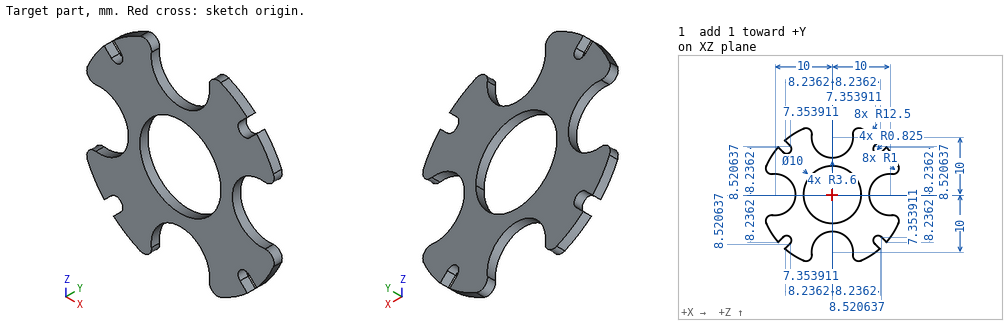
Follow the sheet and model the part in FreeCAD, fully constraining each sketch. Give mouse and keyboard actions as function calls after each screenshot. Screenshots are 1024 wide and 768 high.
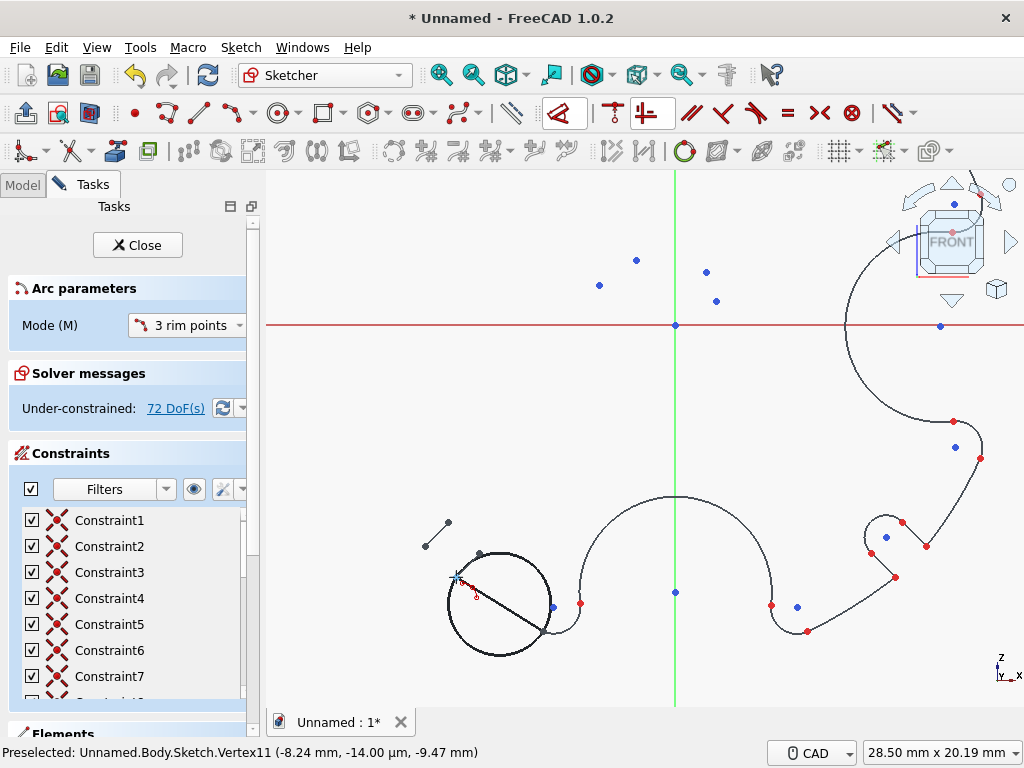
scroll(498, 606, up, 7)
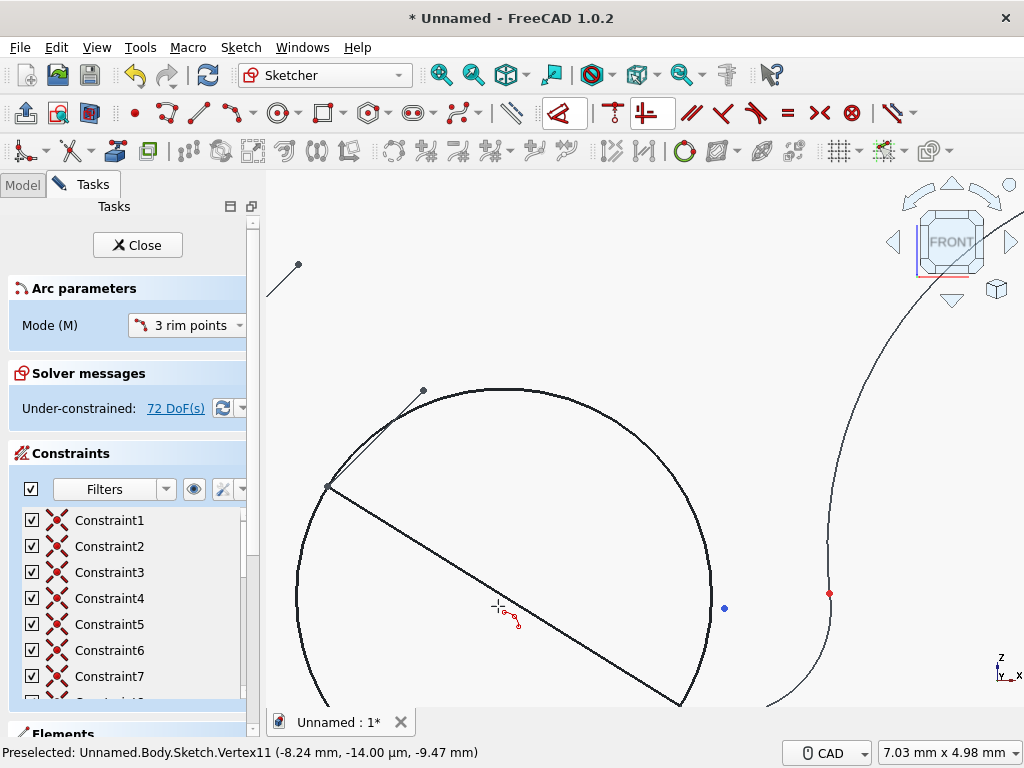
click(496, 605)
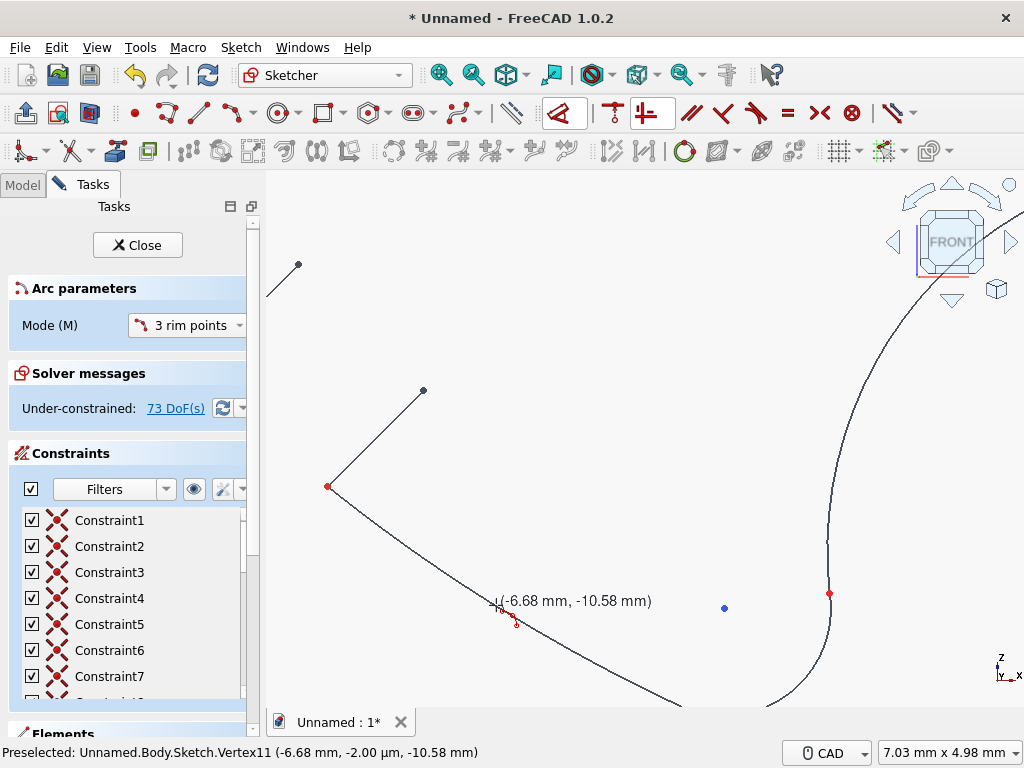
scroll(476, 591, down, 10)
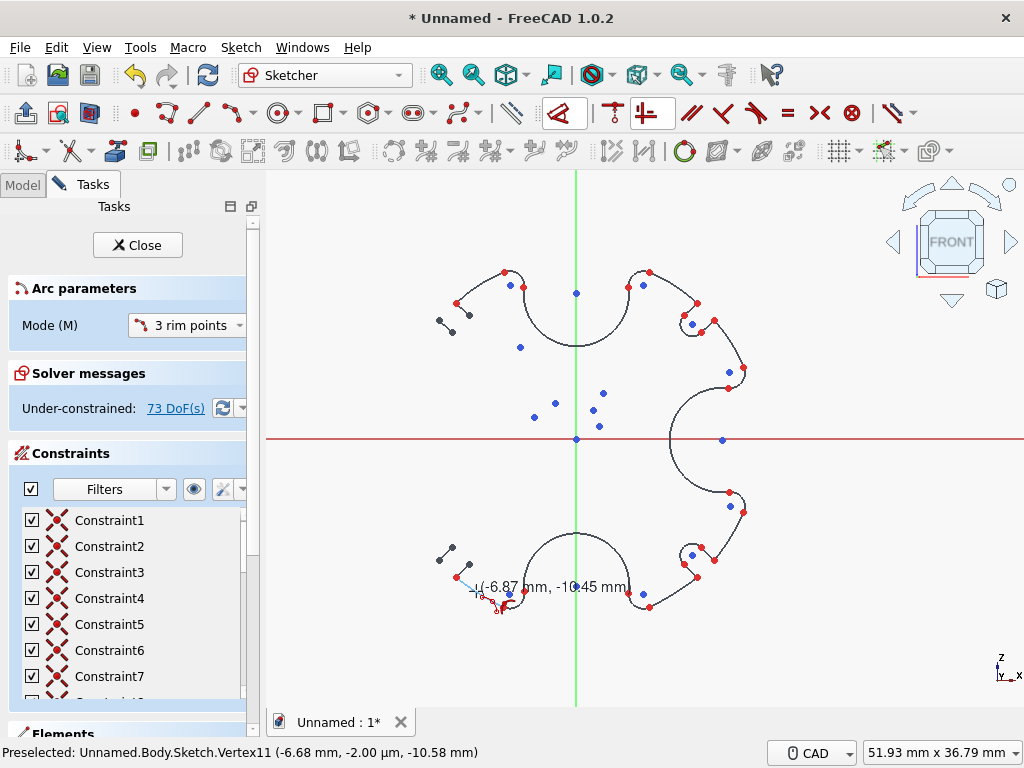
scroll(469, 564, up, 3)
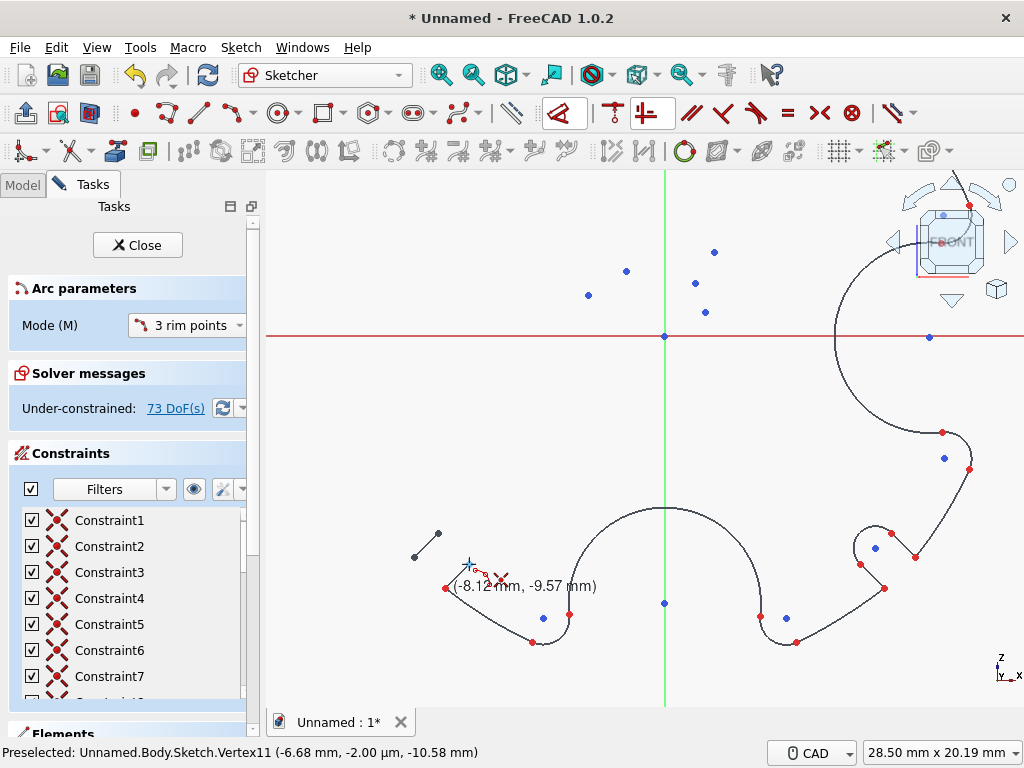
click(469, 564)
click(438, 533)
click(469, 532)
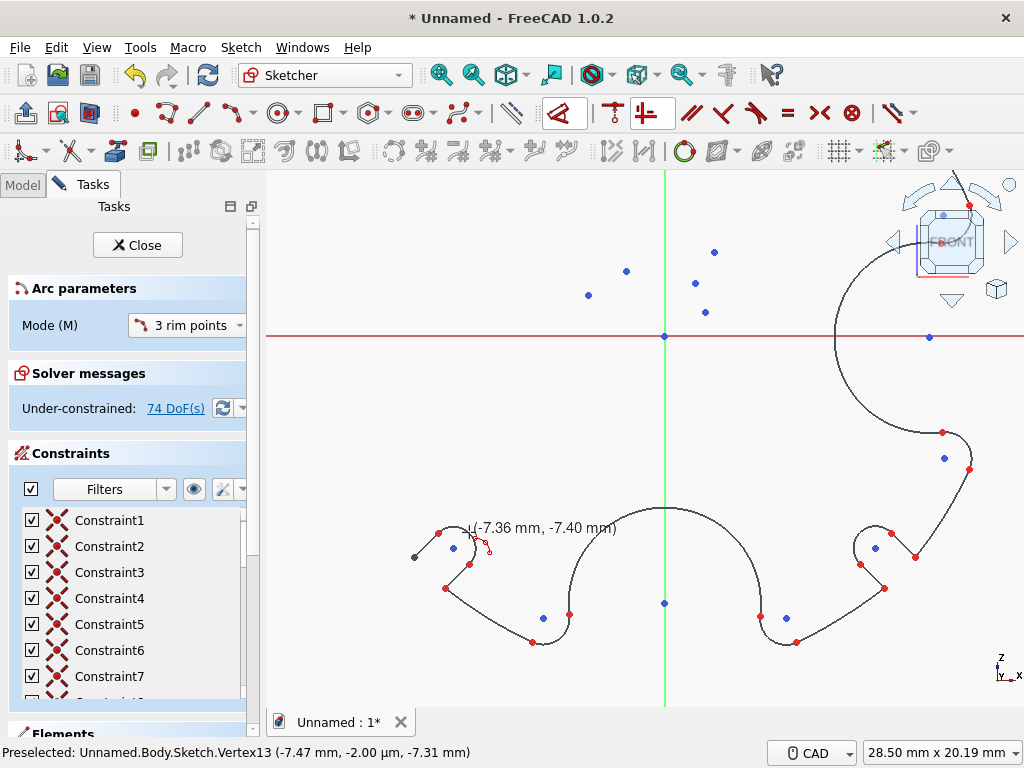
click(414, 557)
click(360, 468)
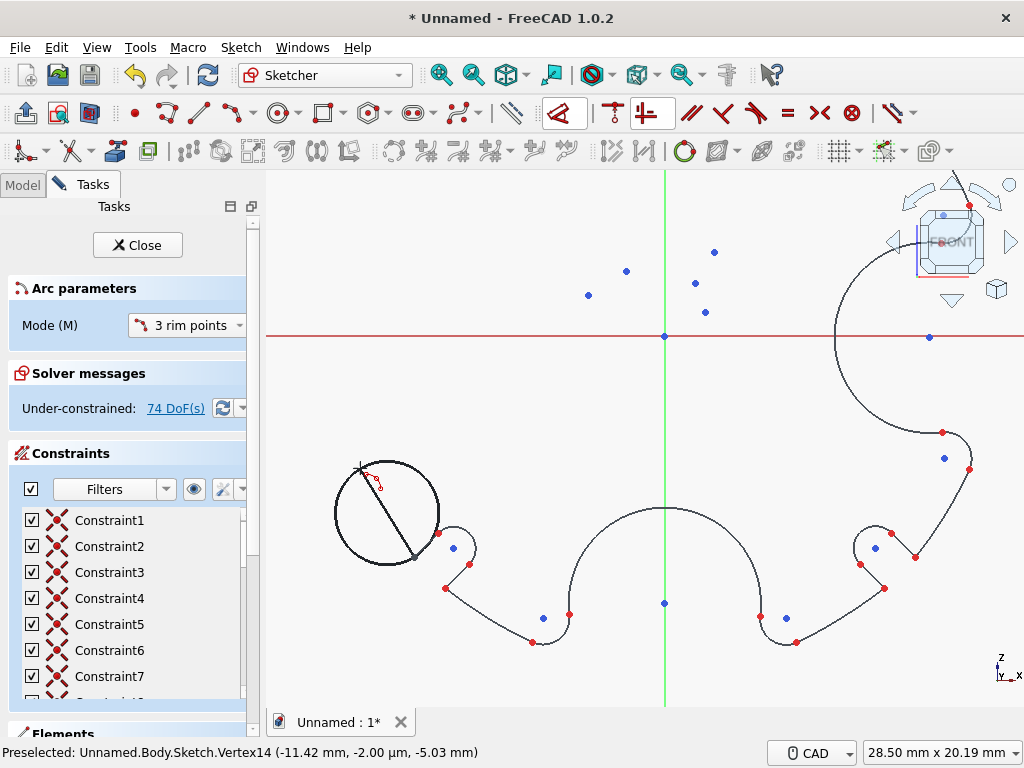
scroll(384, 514, up, 7)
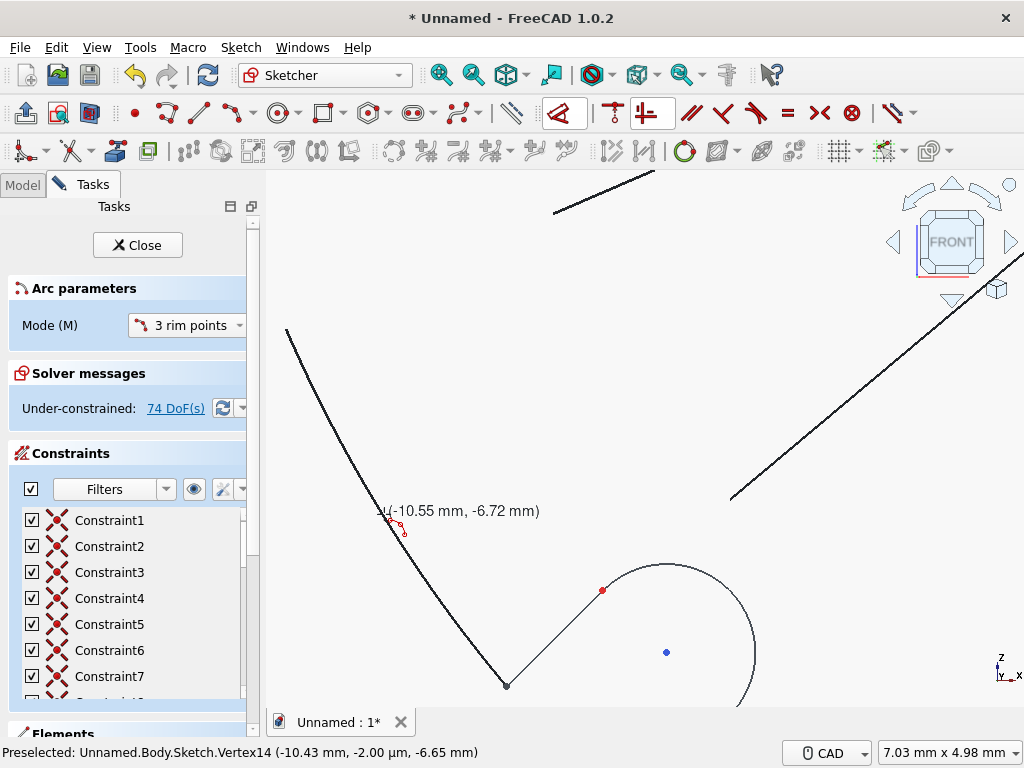
click(382, 512)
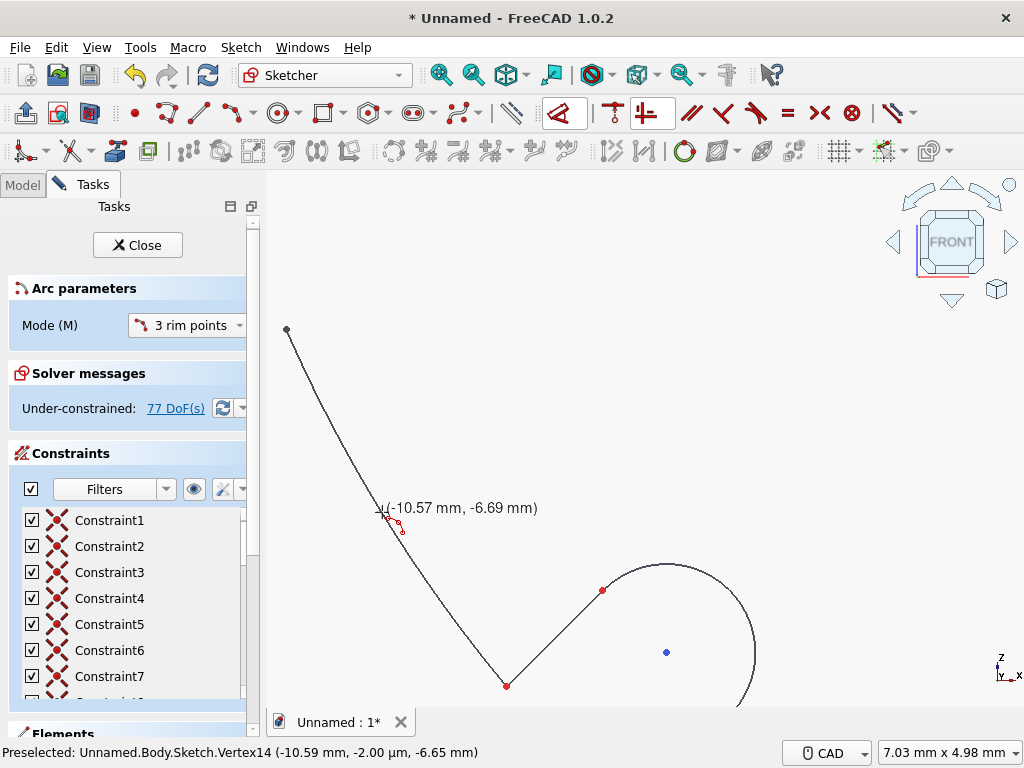
scroll(429, 540, down, 10)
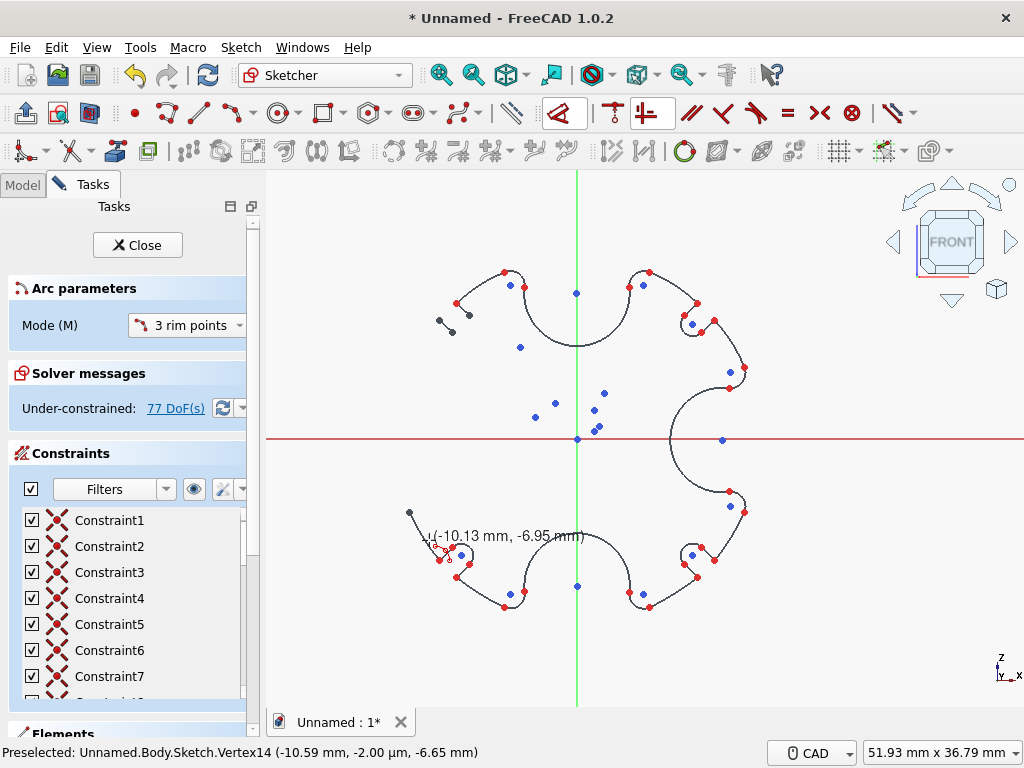
click(410, 512)
click(425, 491)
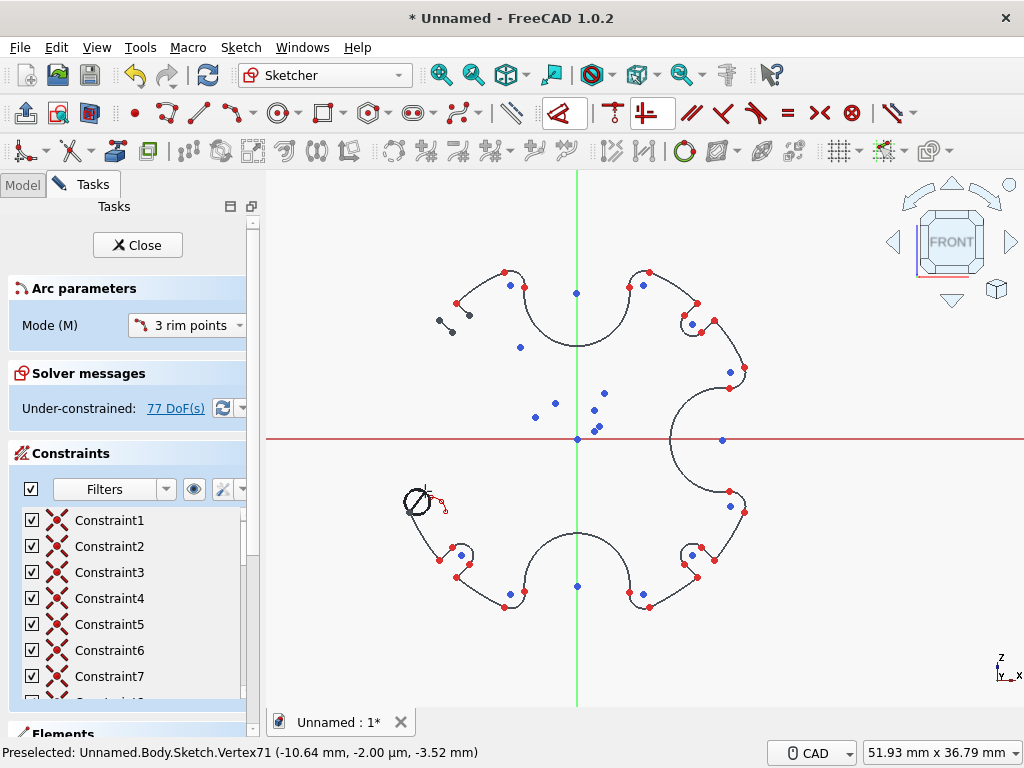
scroll(411, 497, up, 4)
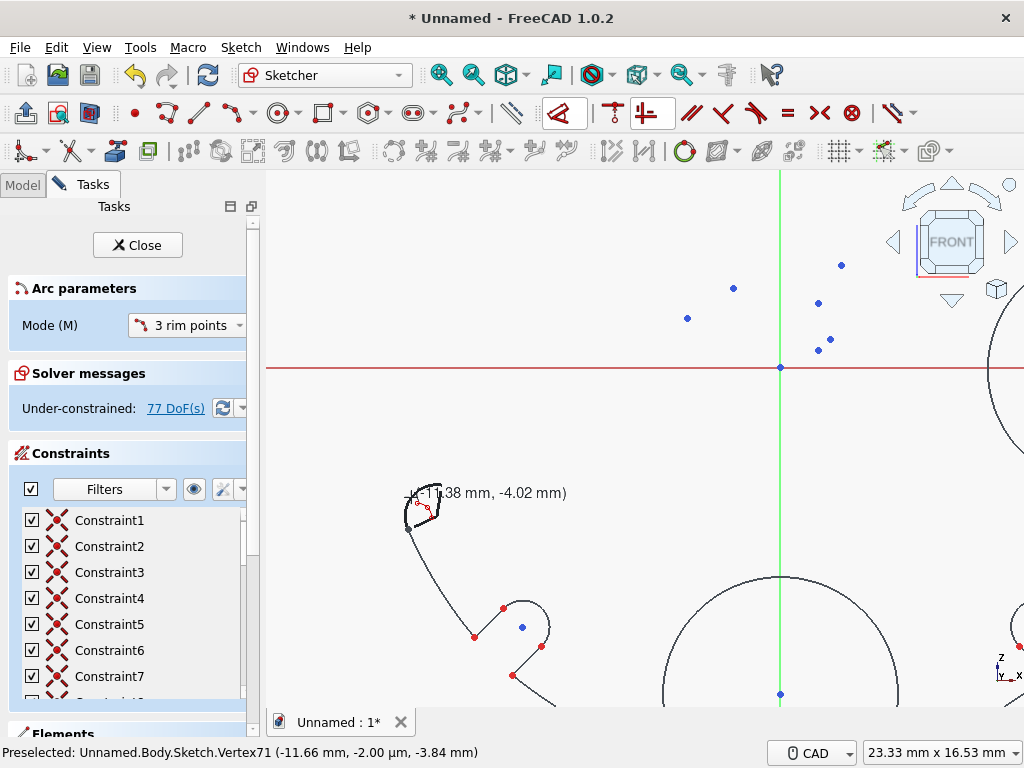
click(411, 497)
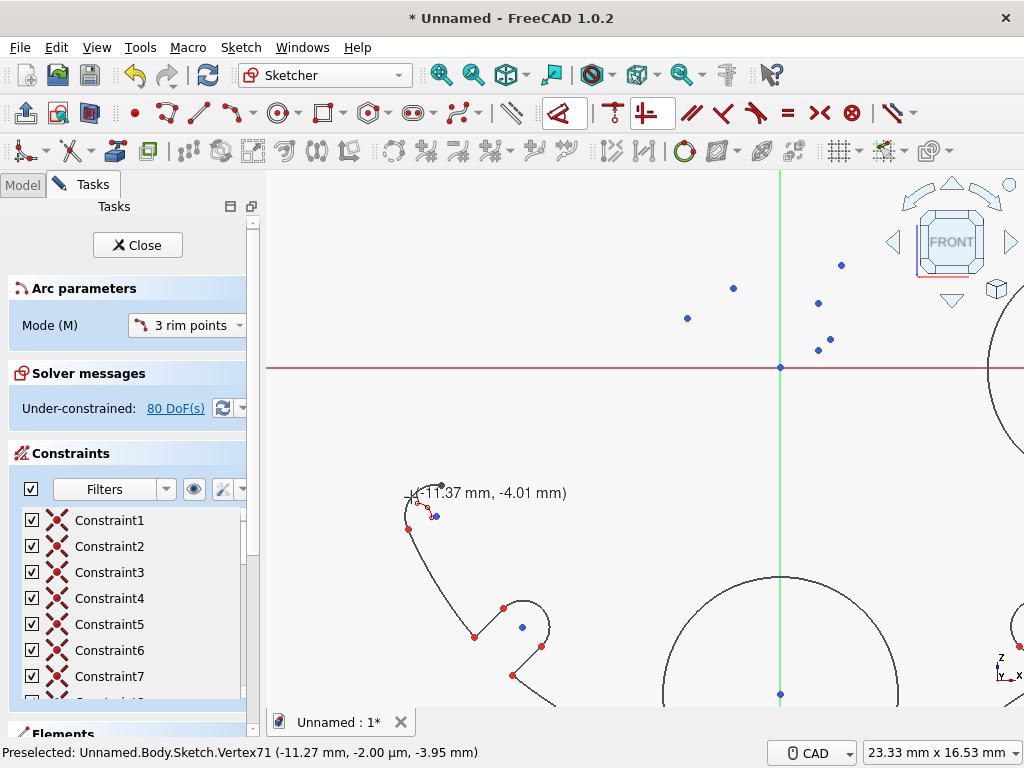
click(442, 485)
click(441, 252)
click(566, 407)